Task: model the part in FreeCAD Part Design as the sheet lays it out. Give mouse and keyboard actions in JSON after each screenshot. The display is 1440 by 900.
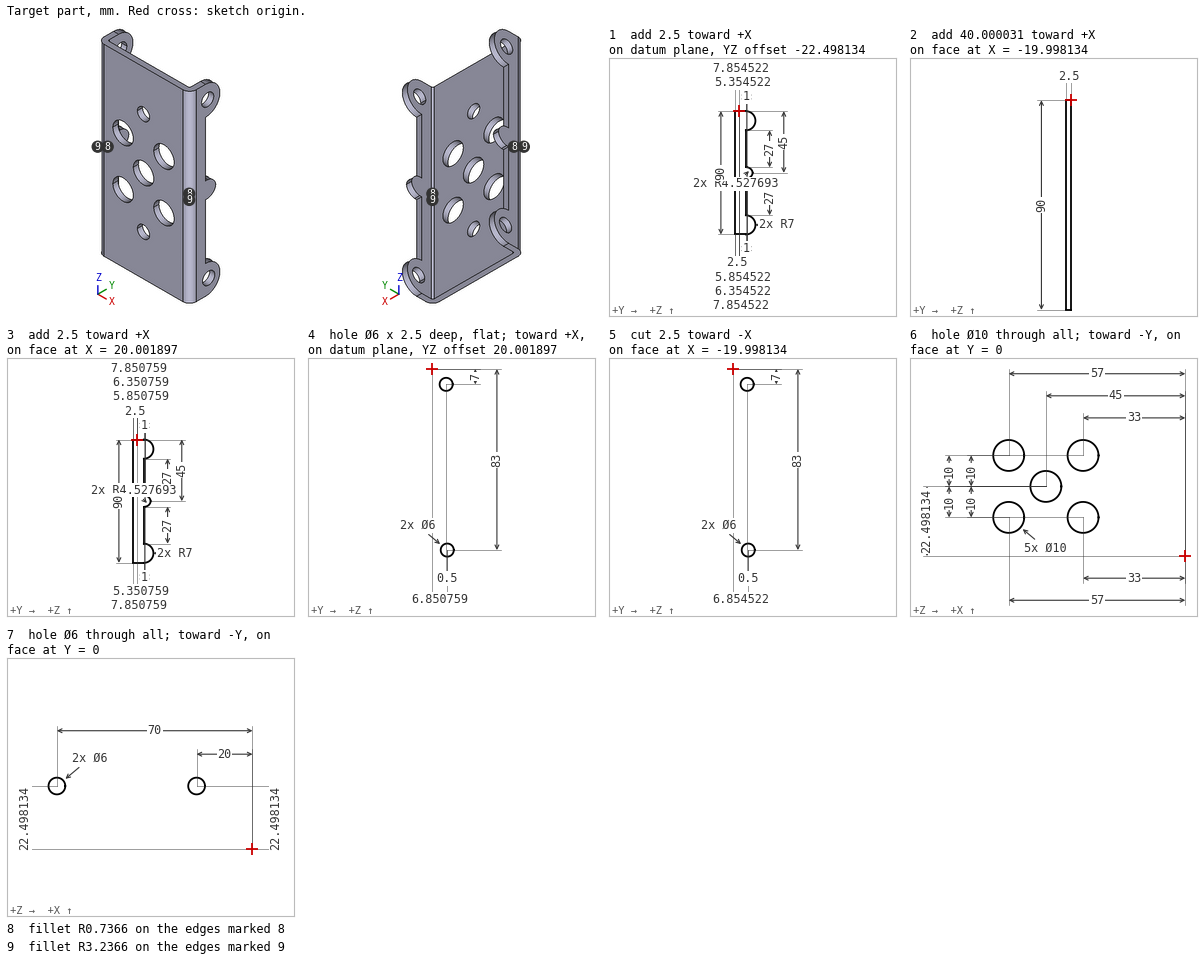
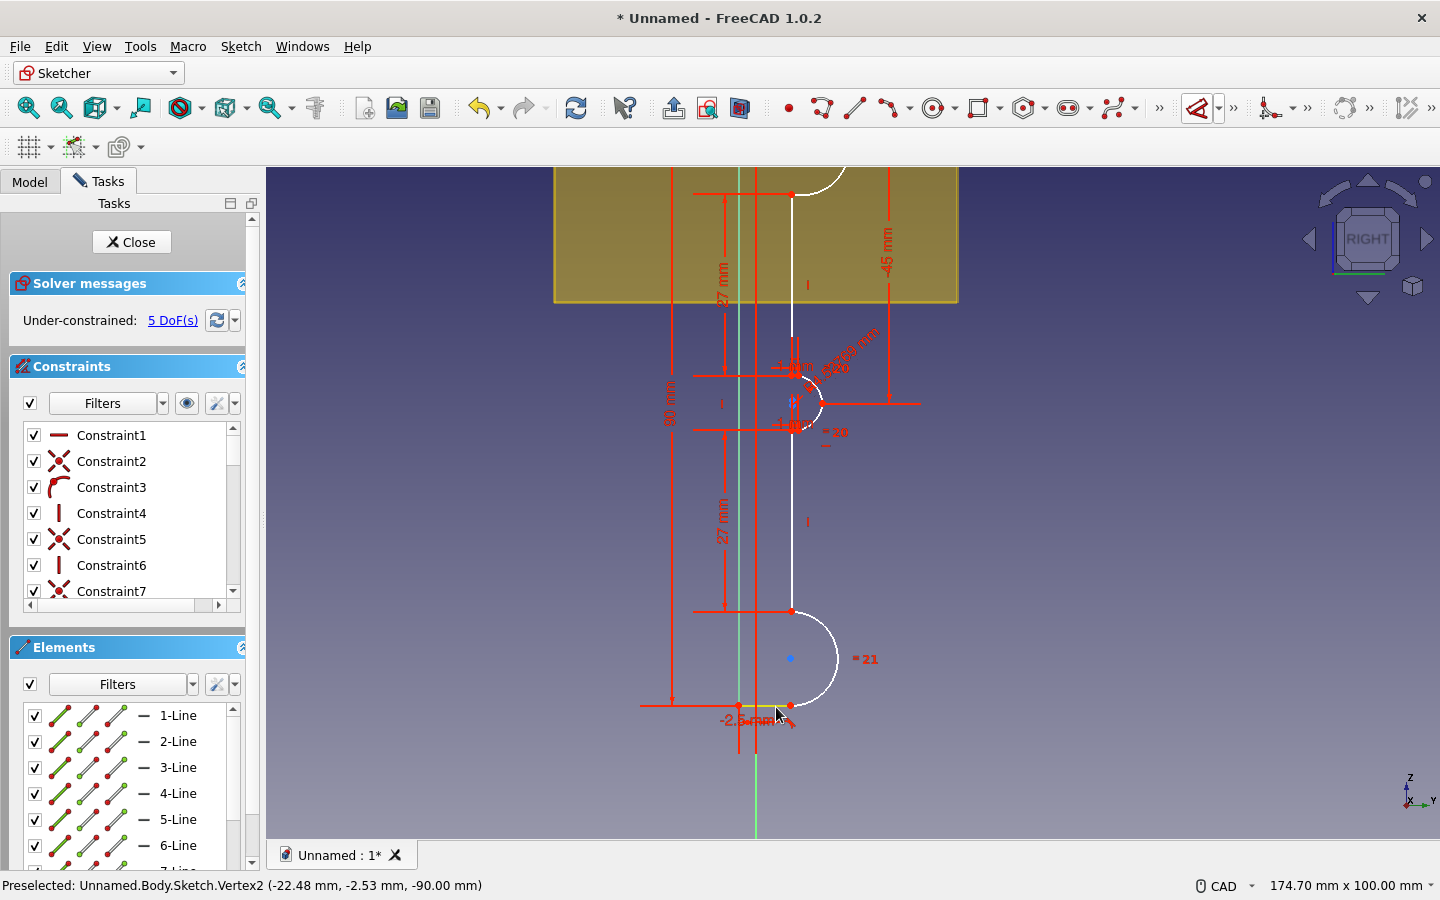
{"action": "left_click", "coordinate": [775, 706]}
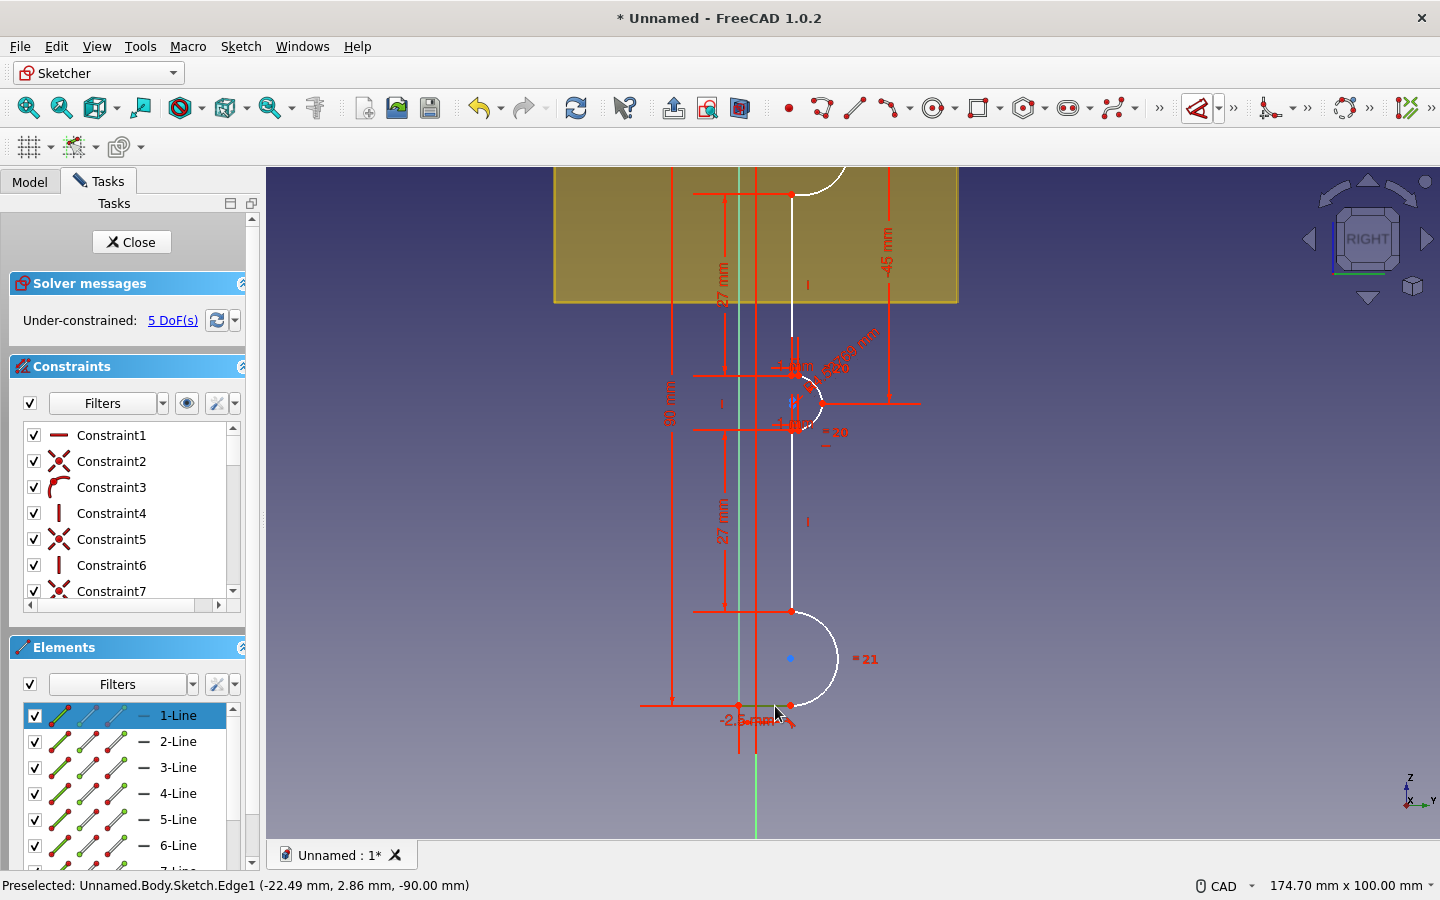
{"action": "left_click", "coordinate": [1218, 108]}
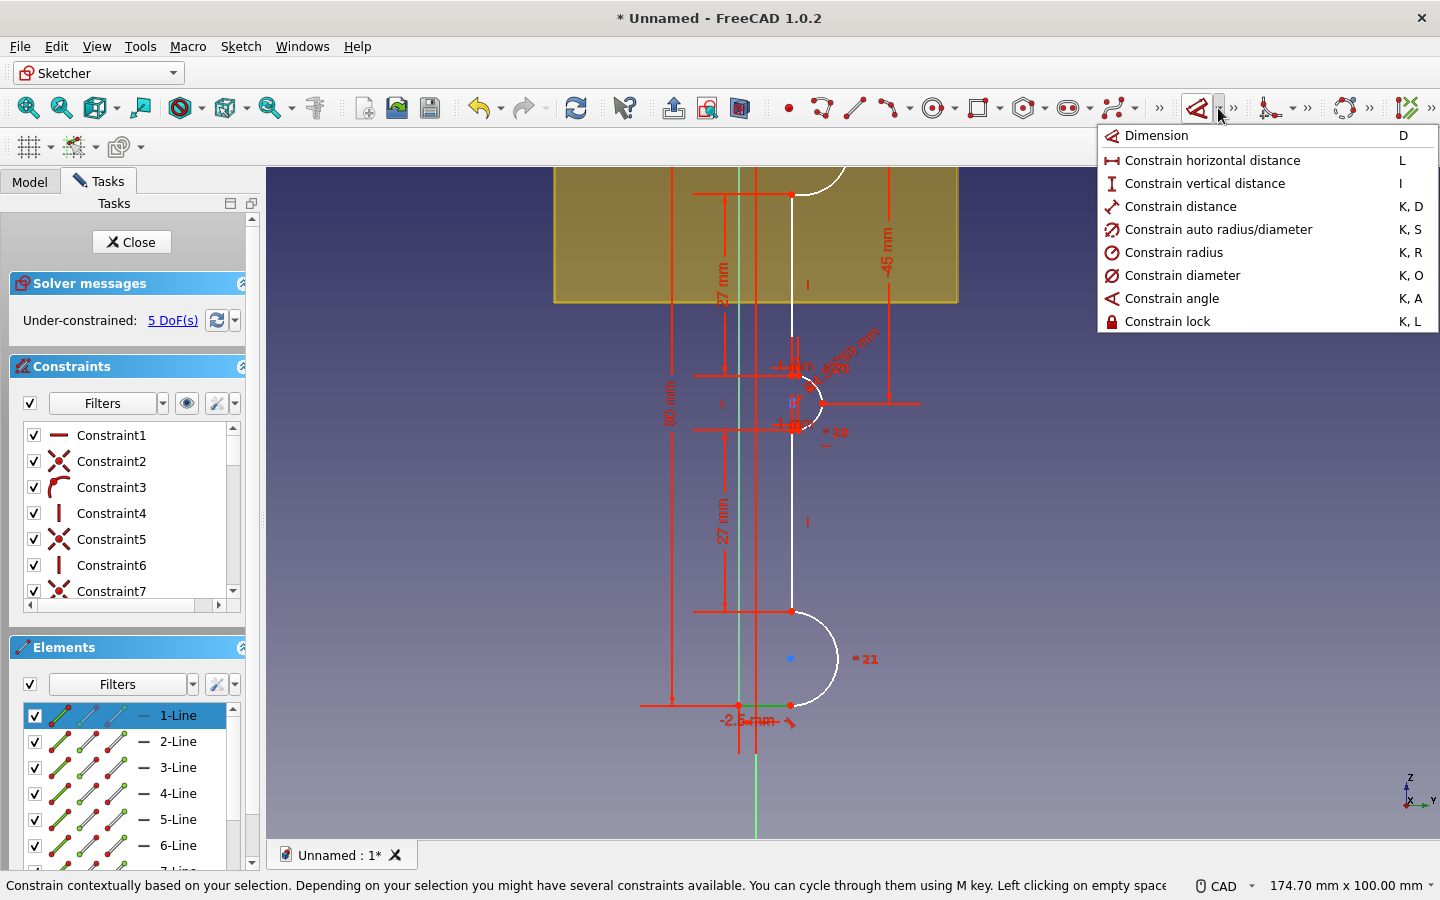
{"action": "left_click", "coordinate": [1268, 160]}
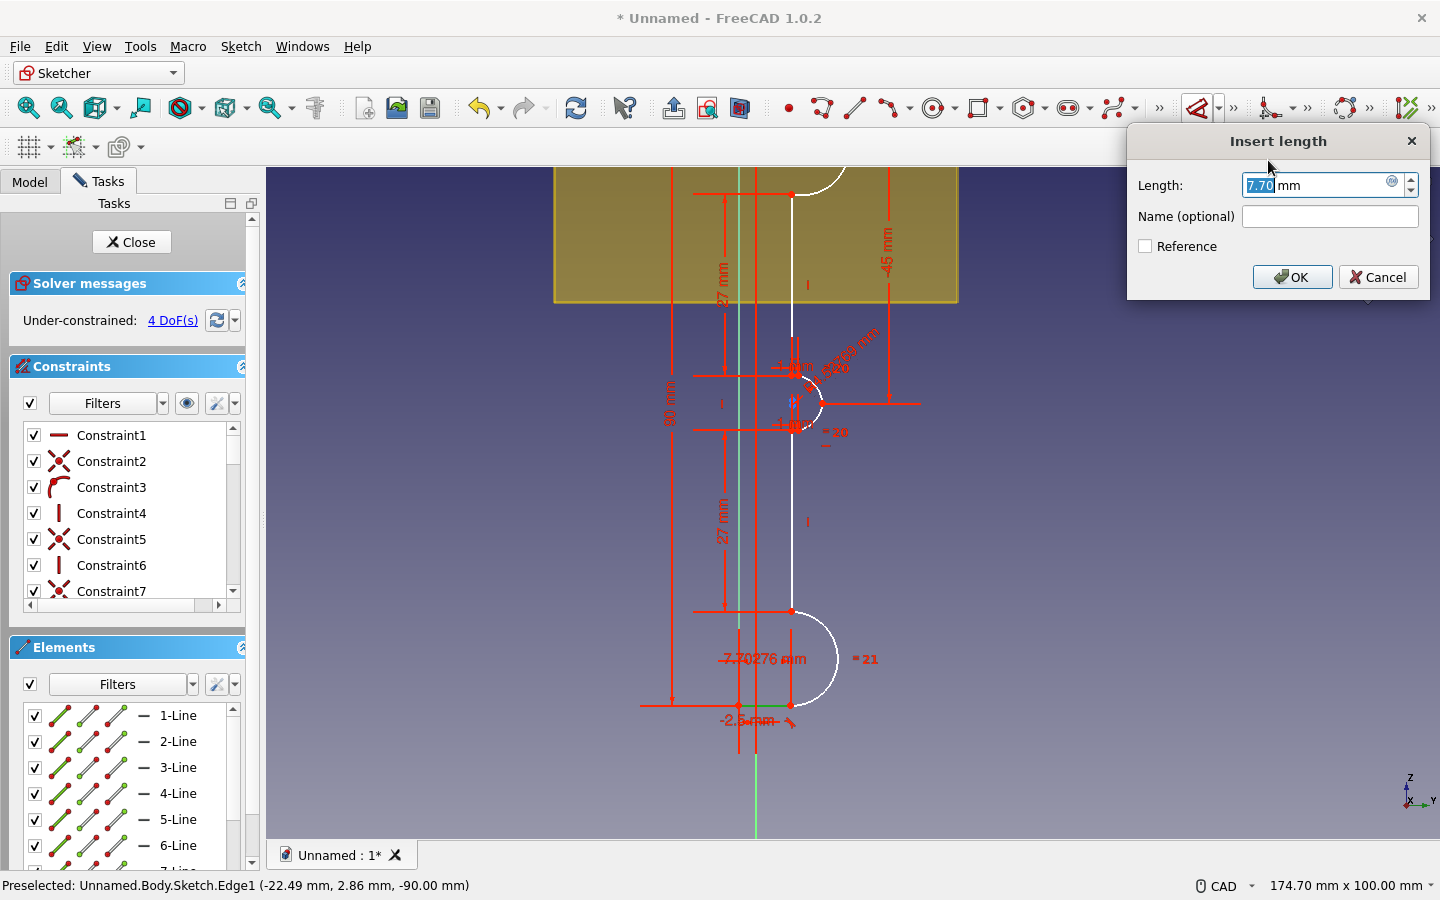
{"action": "type", "text": "7.854522"}
{"action": "key", "text": "Return"}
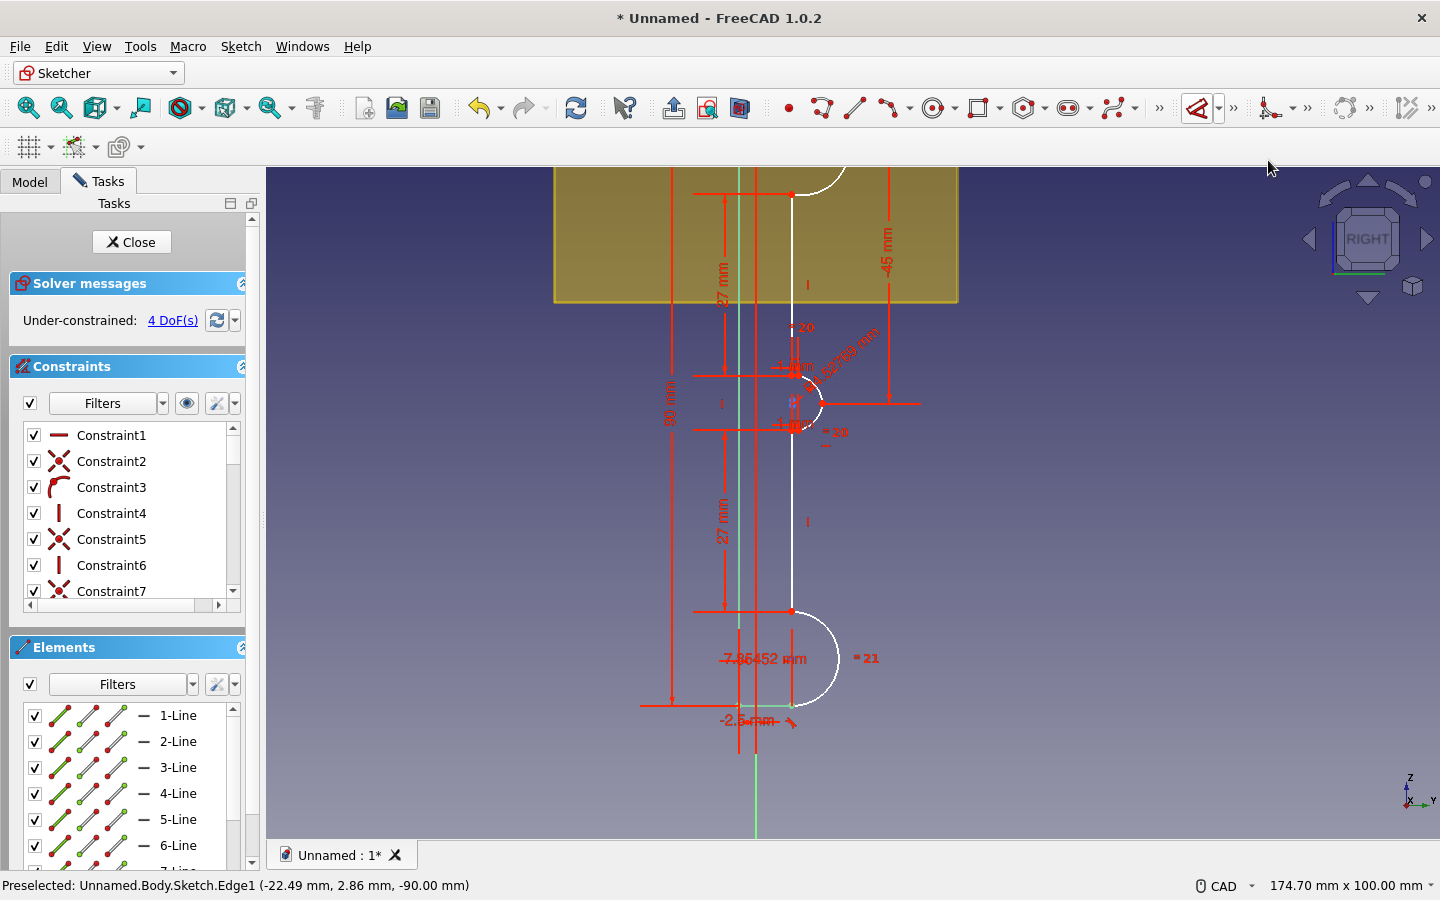
{"action": "scroll", "coordinate": [776, 705], "scroll_direction": "down", "scroll_amount": 2}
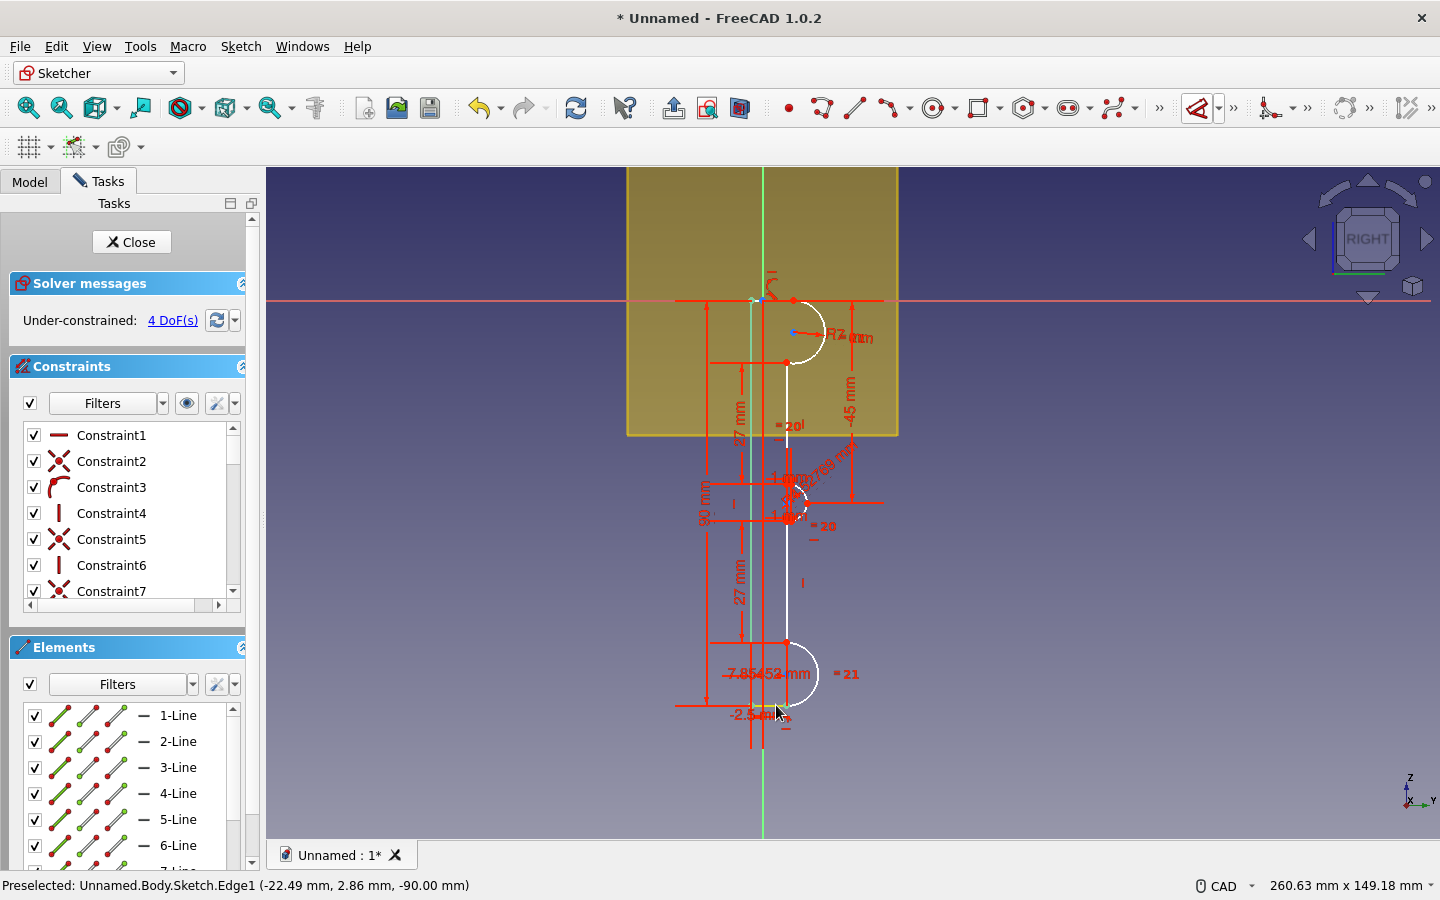
{"action": "left_click", "coordinate": [781, 301]}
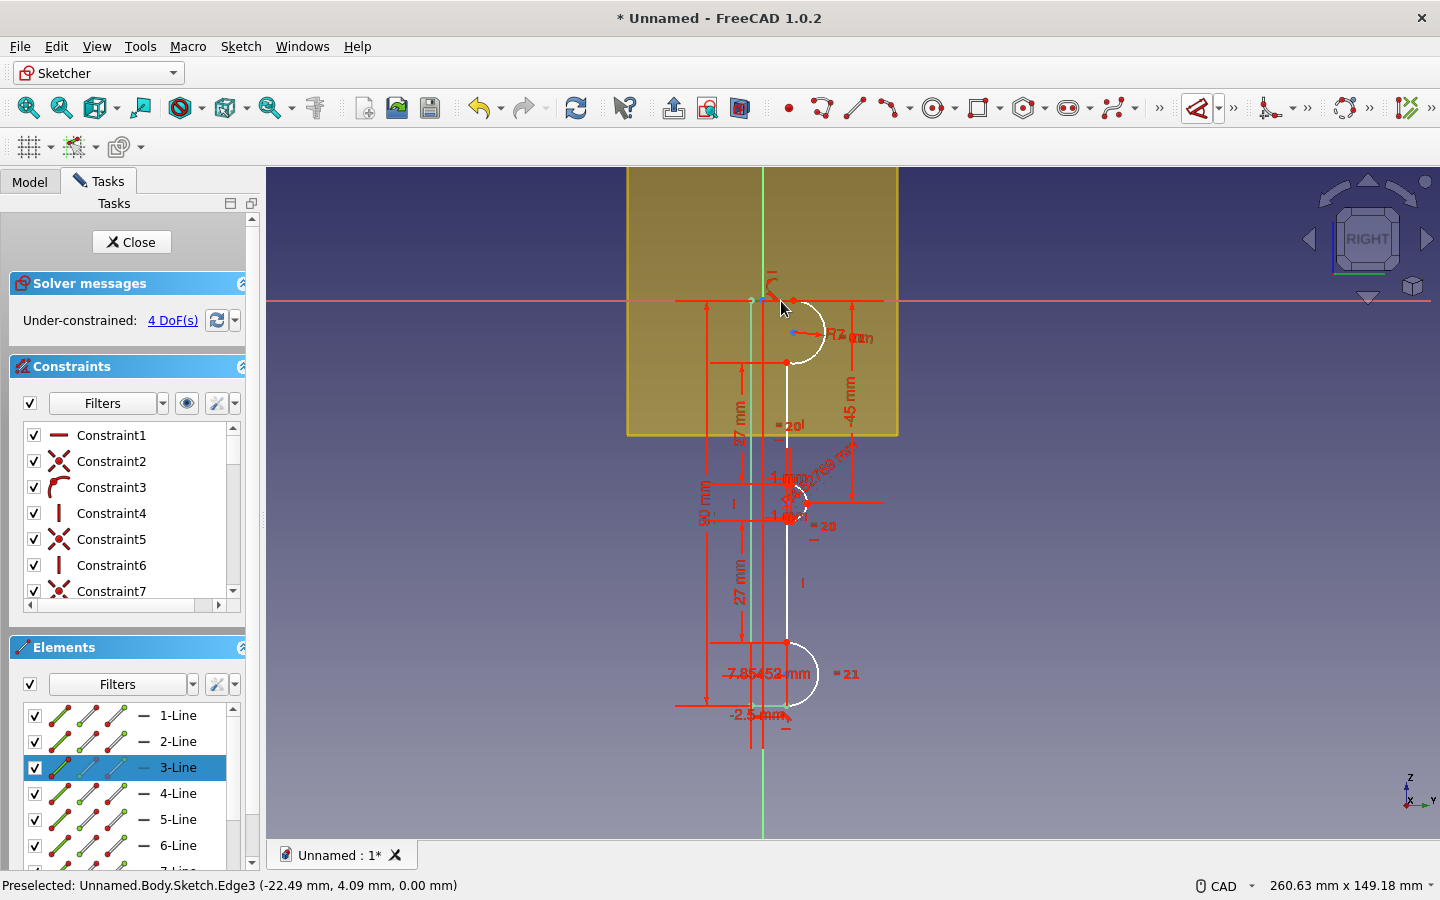
{"action": "key", "text": "l"}